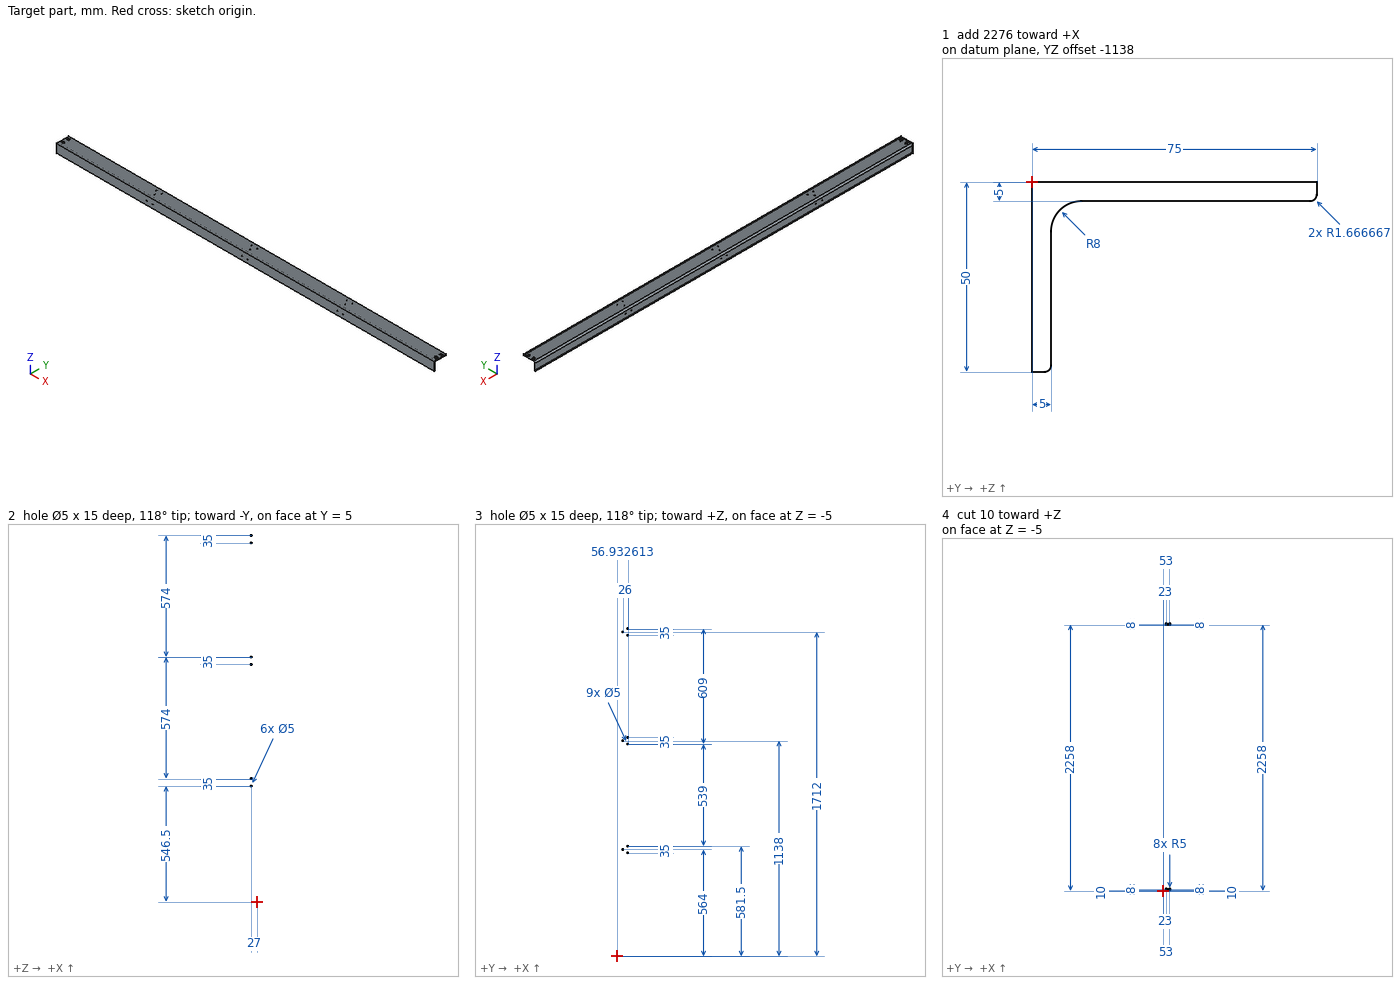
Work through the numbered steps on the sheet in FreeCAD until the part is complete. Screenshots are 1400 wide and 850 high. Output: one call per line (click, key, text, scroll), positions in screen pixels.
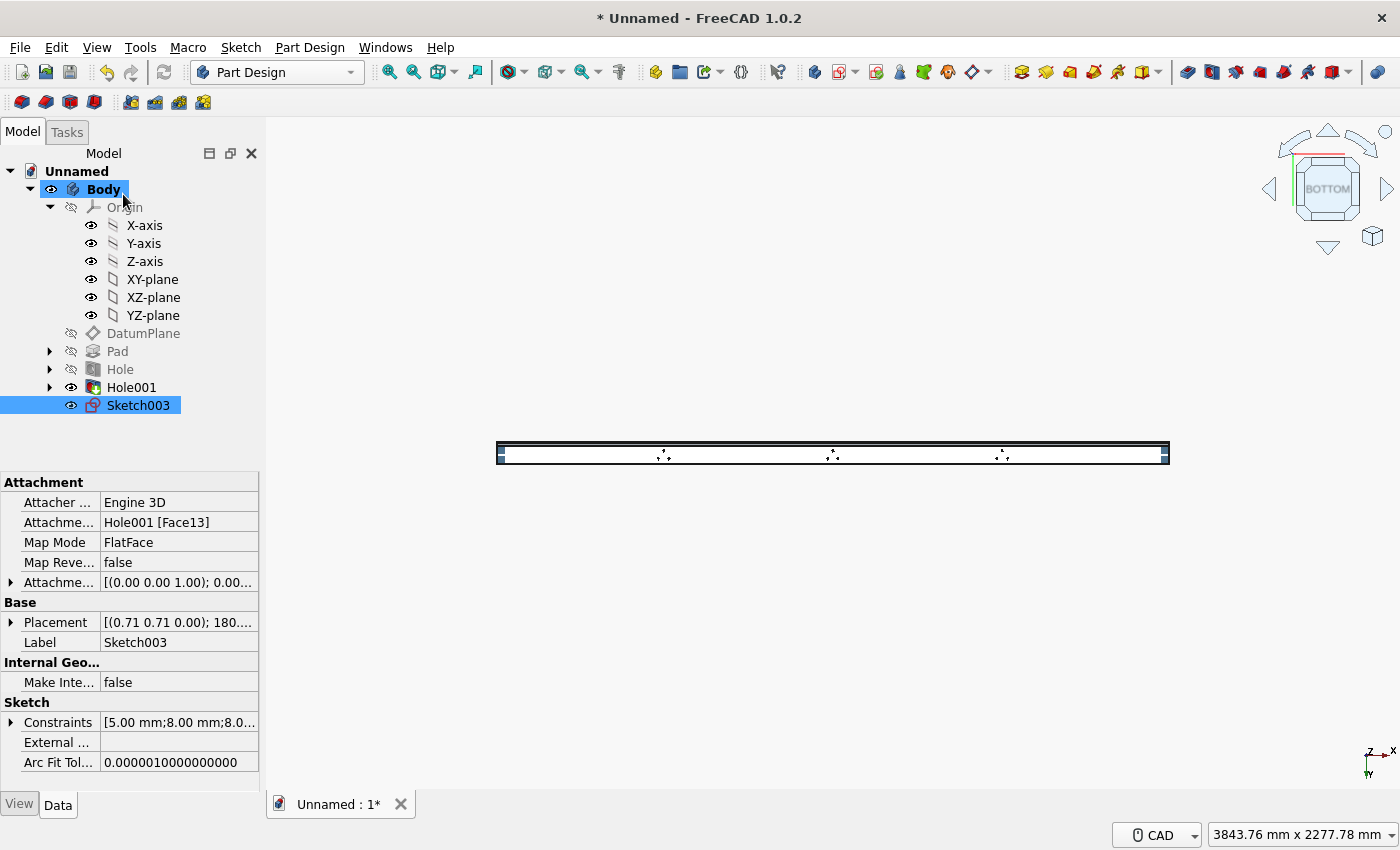
click(1188, 72)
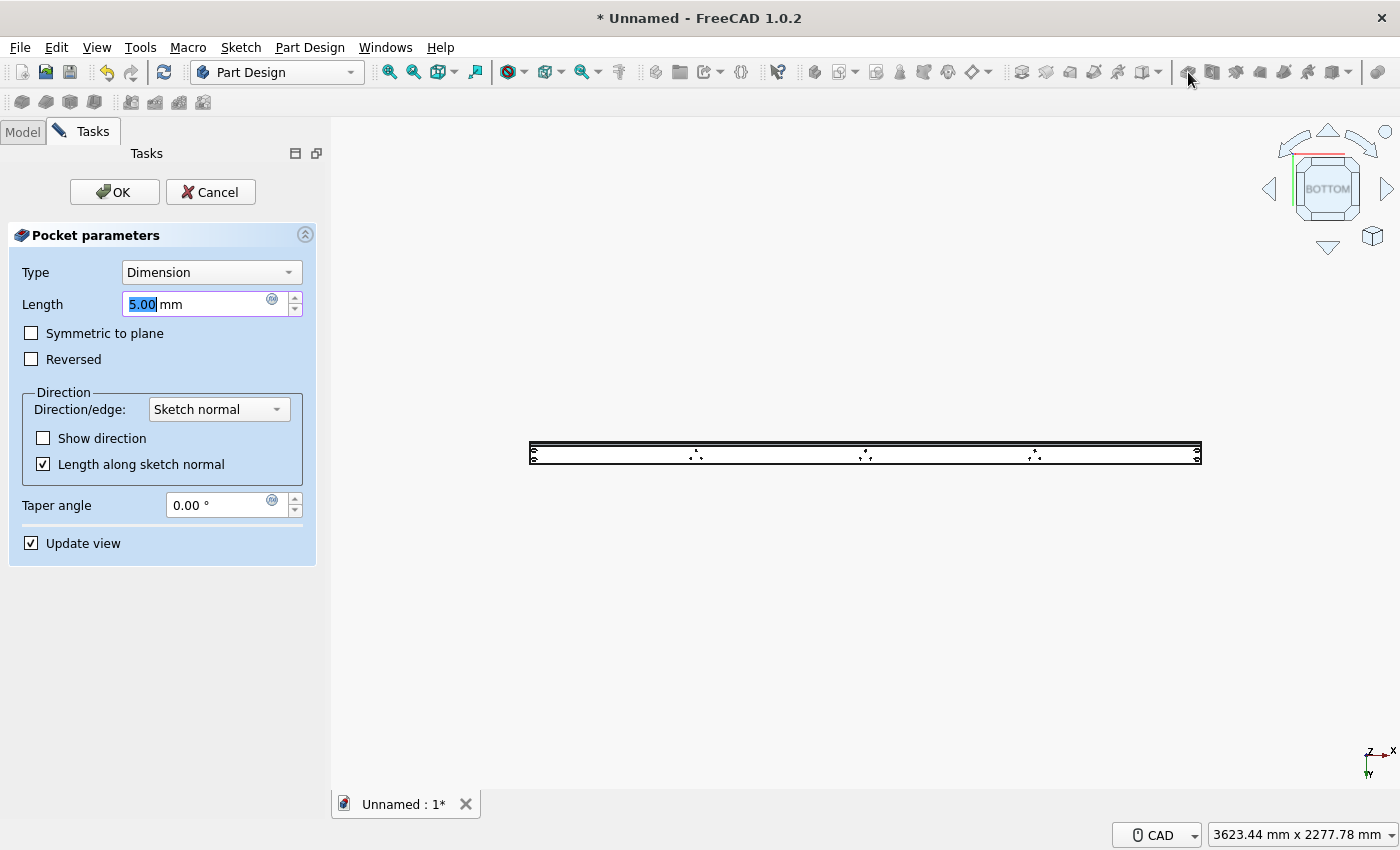
text(10)
key(Tab)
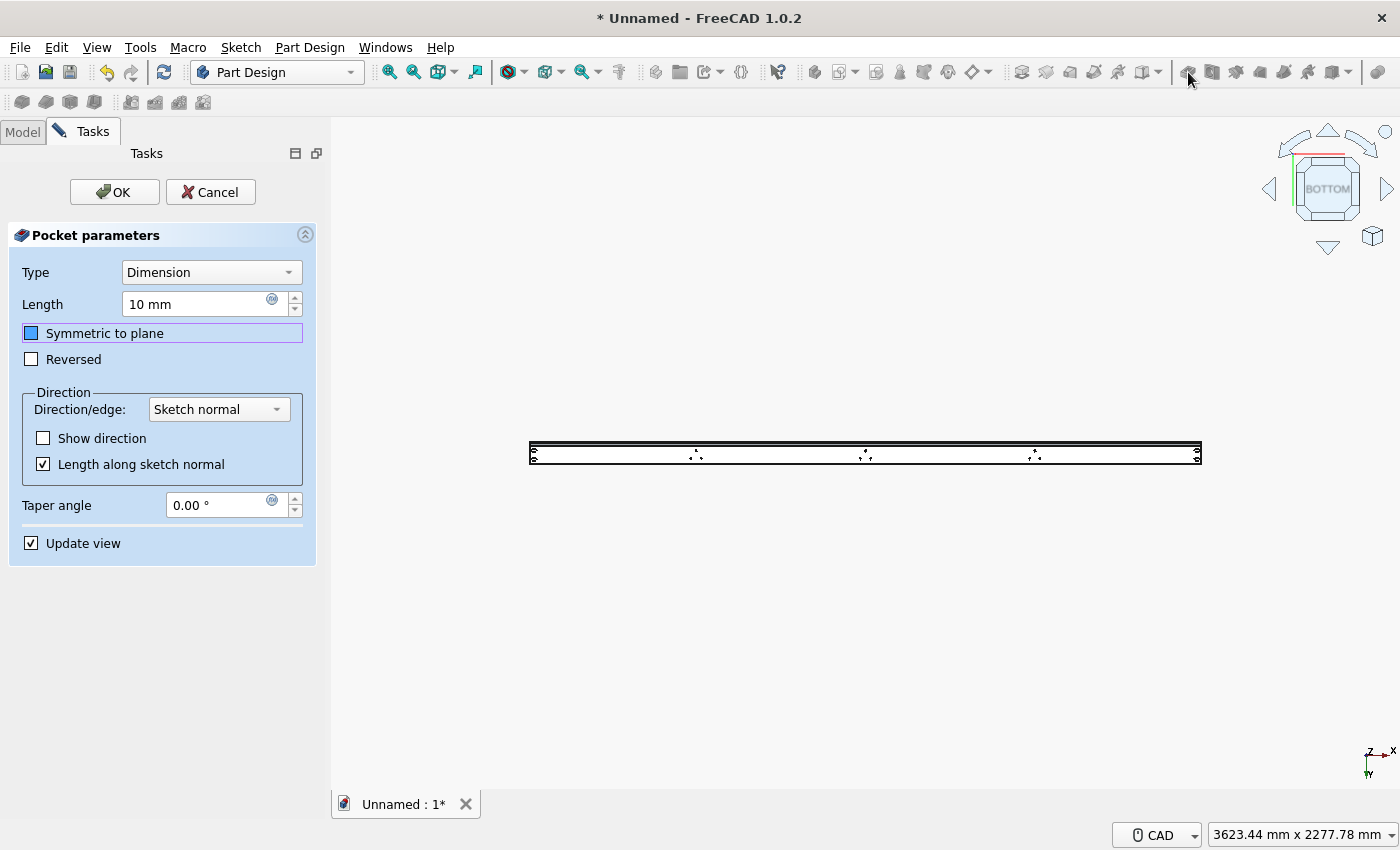
click(115, 192)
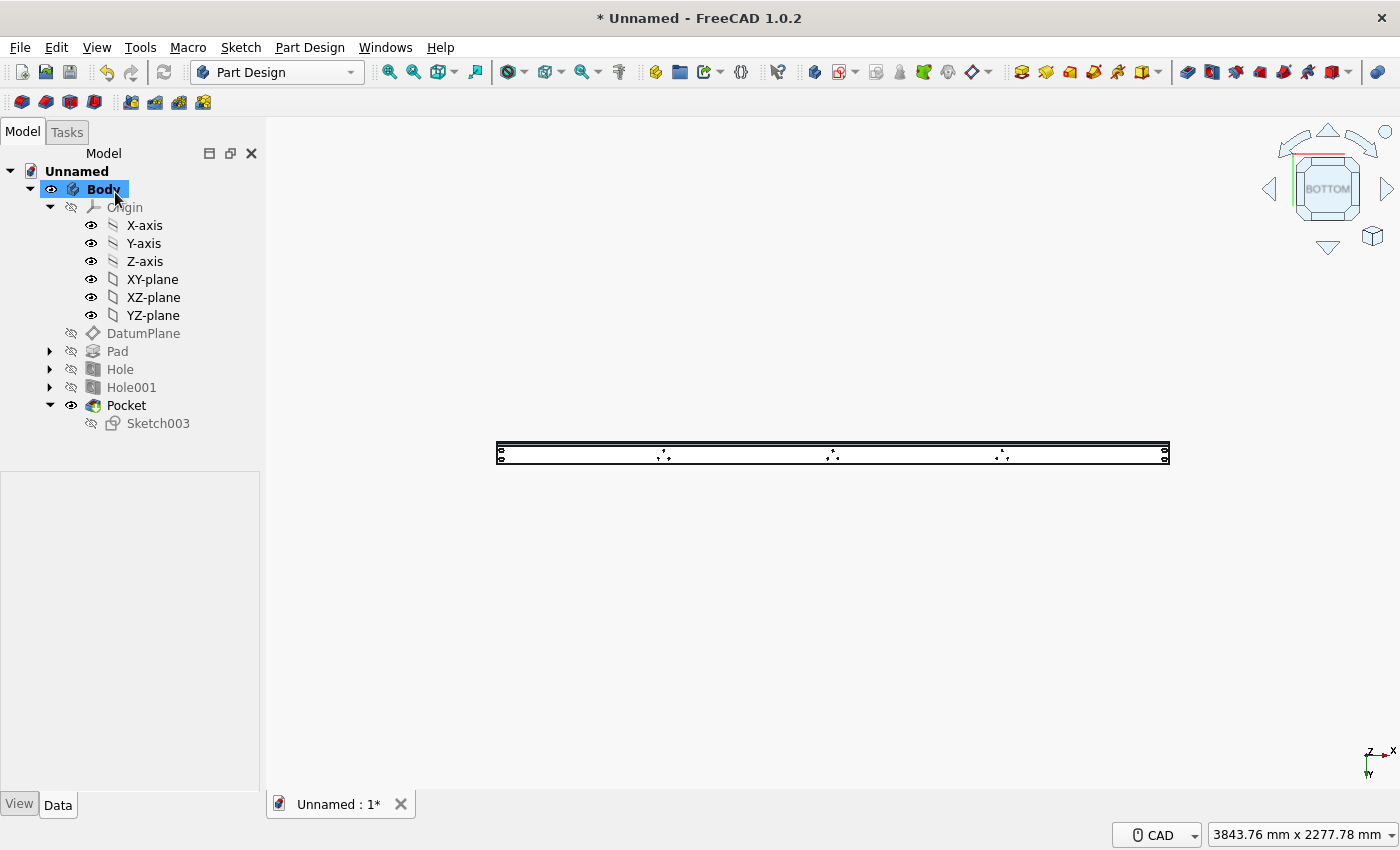
key(0)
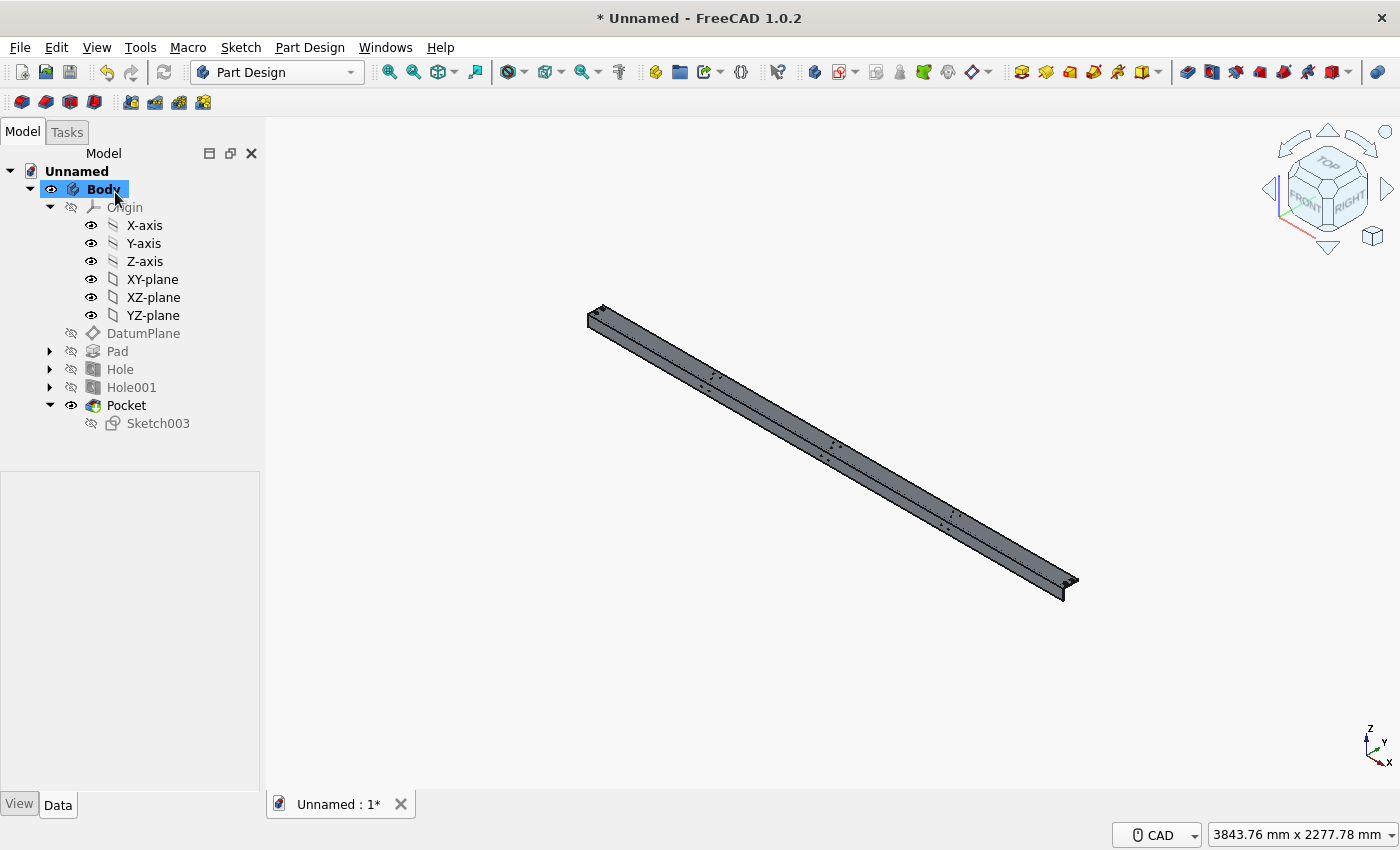
click(390, 72)